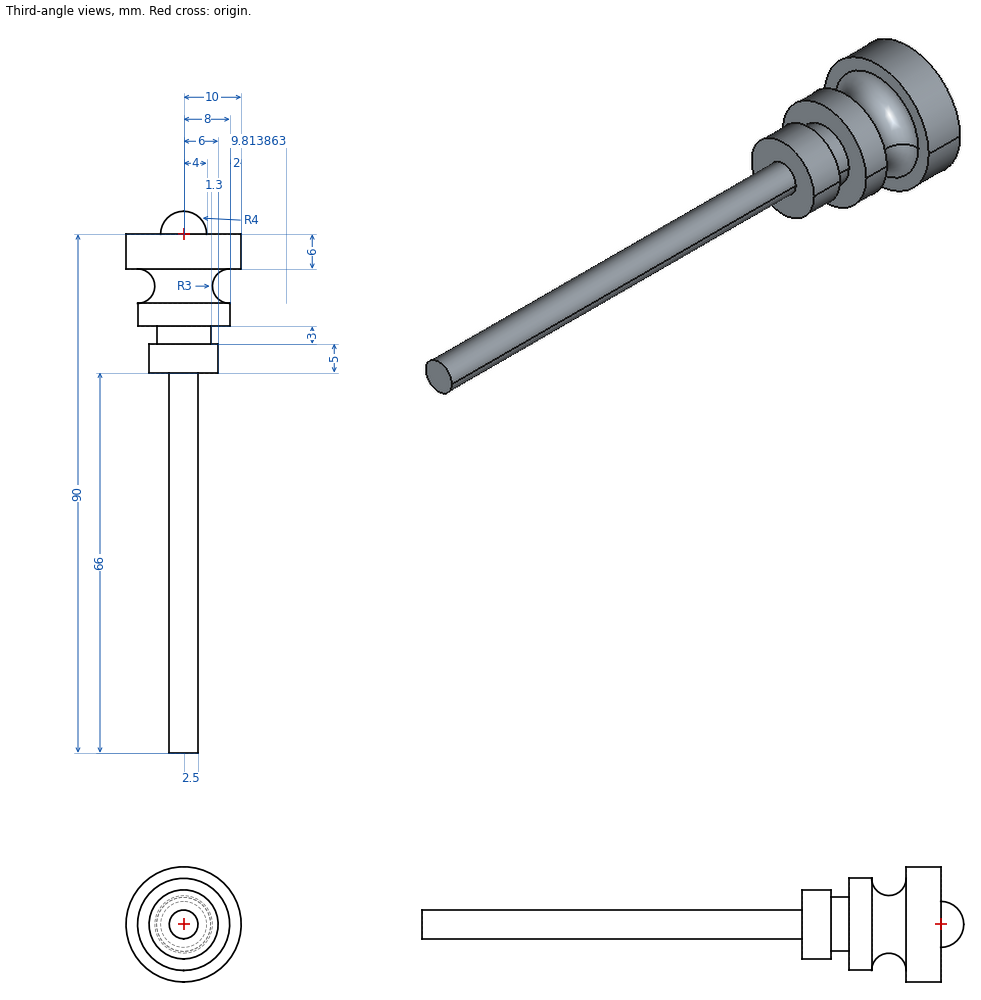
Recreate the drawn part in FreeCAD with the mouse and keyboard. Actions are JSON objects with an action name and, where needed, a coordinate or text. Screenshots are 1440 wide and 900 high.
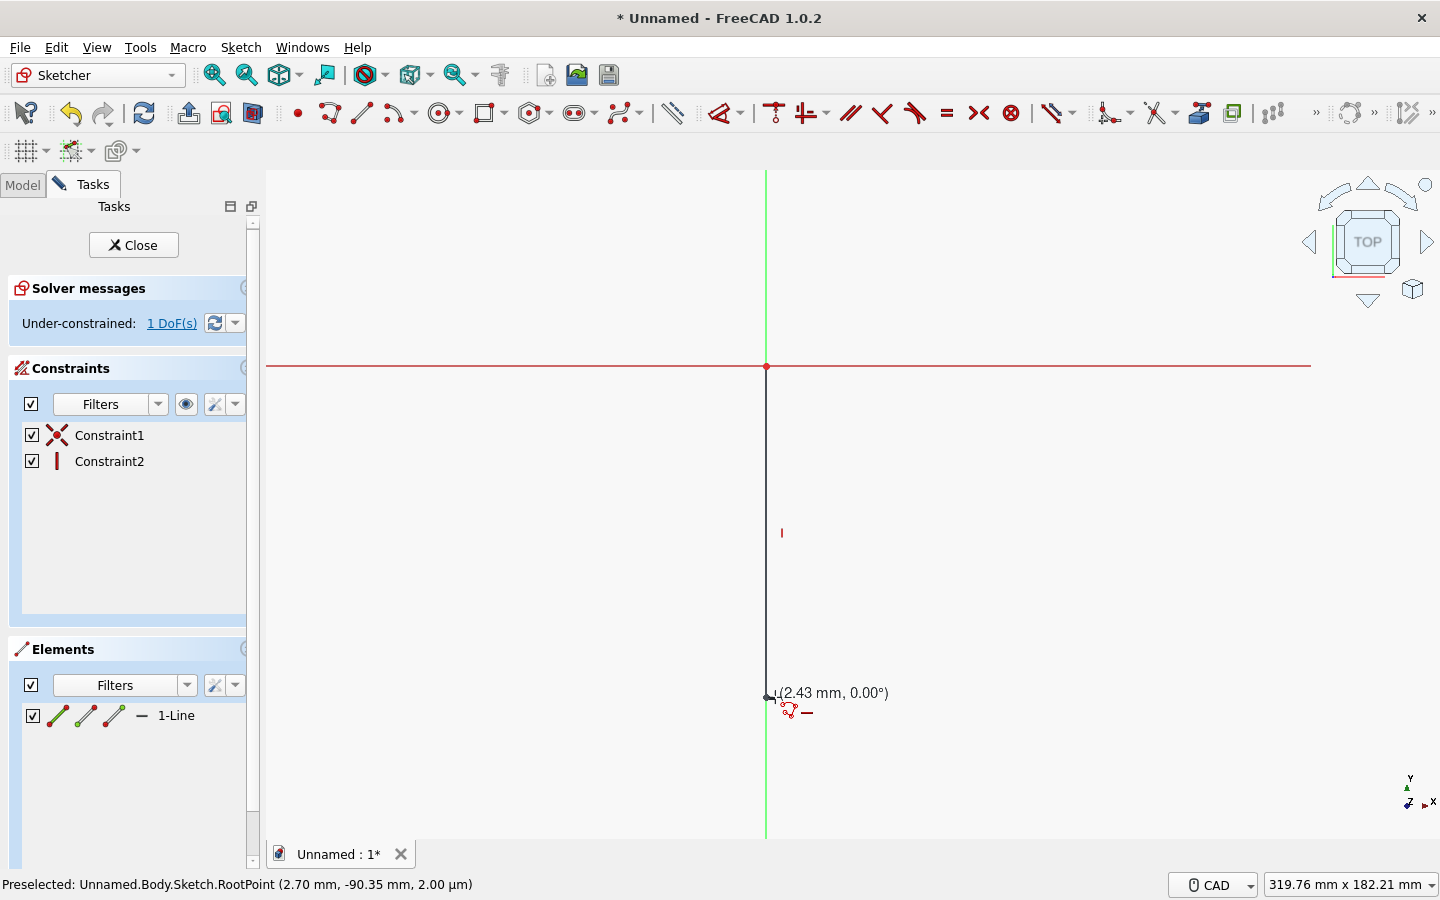
{"action": "scroll", "coordinate": [775, 697], "scroll_direction": "up", "scroll_amount": 3}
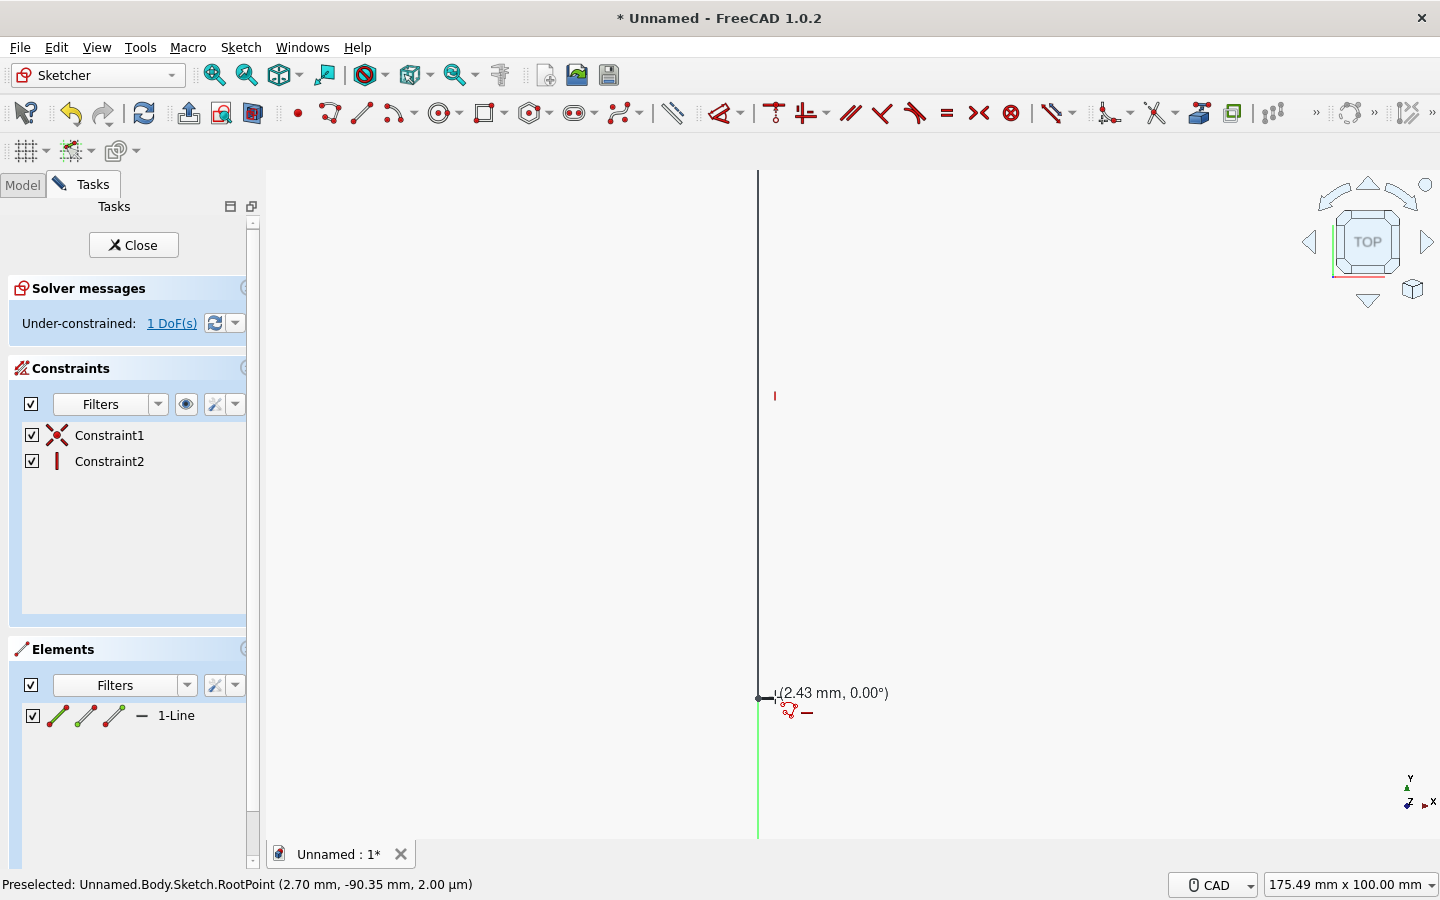
{"action": "left_click", "coordinate": [775, 696]}
{"action": "left_click", "coordinate": [775, 254]}
{"action": "left_click", "coordinate": [799, 254]}
{"action": "left_click", "coordinate": [799, 221]}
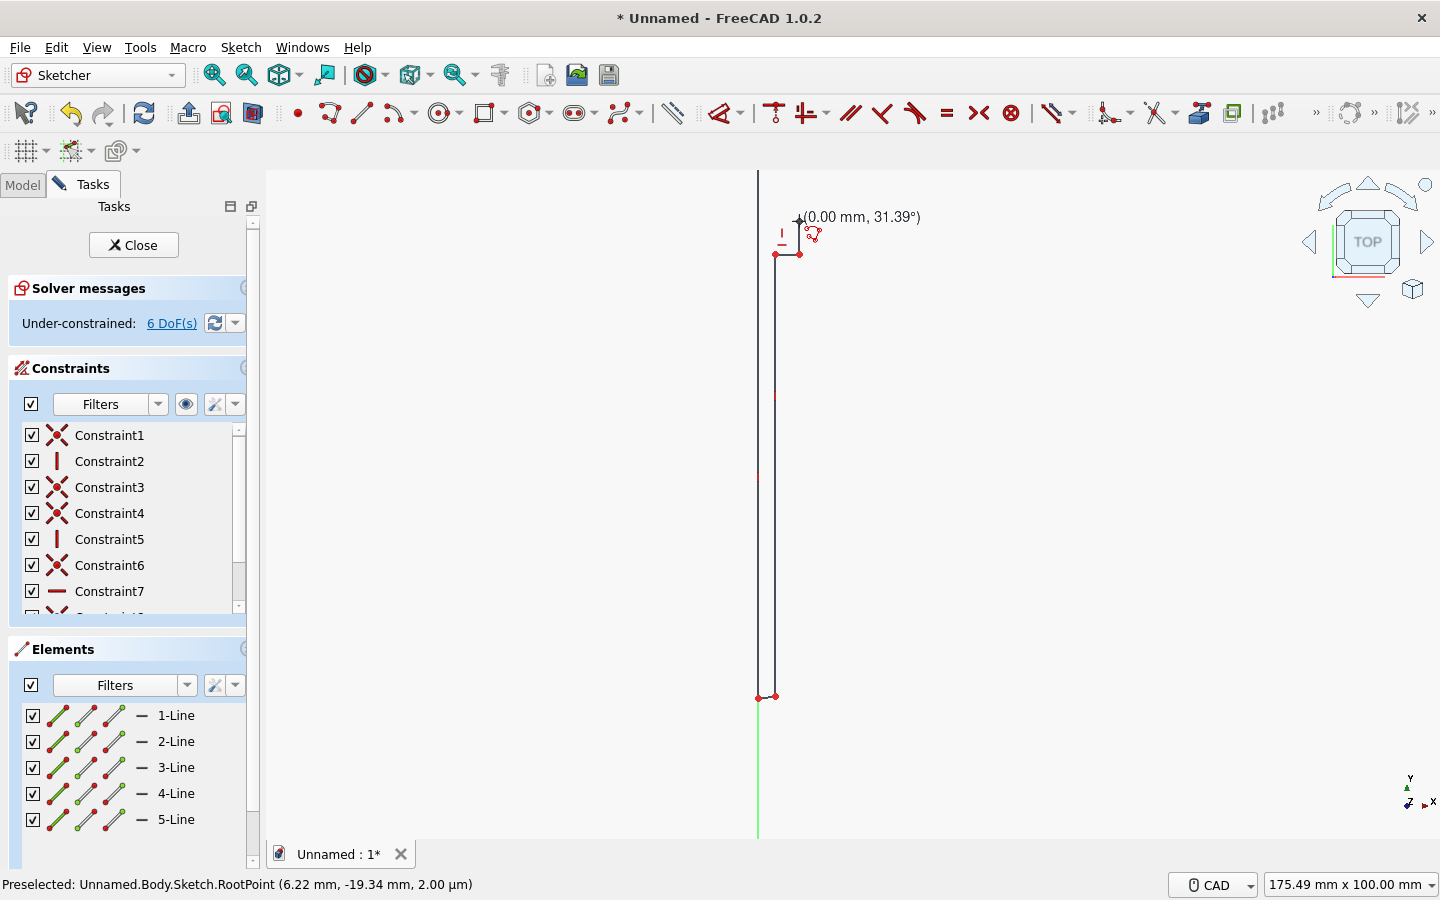
{"action": "scroll", "coordinate": [790, 221], "scroll_direction": "up", "scroll_amount": 4}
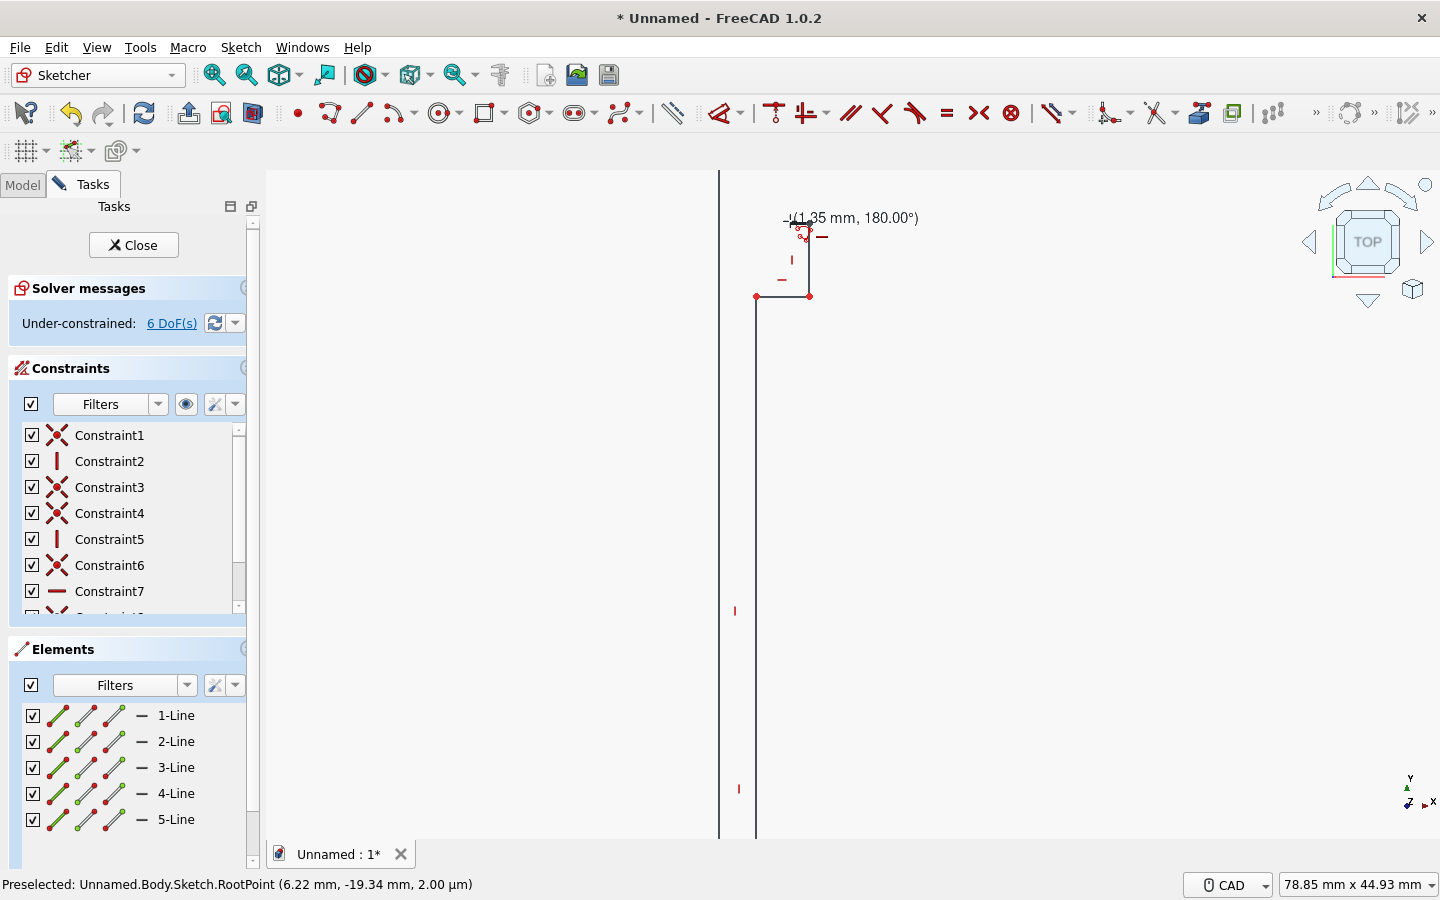
{"action": "left_click", "coordinate": [789, 221]}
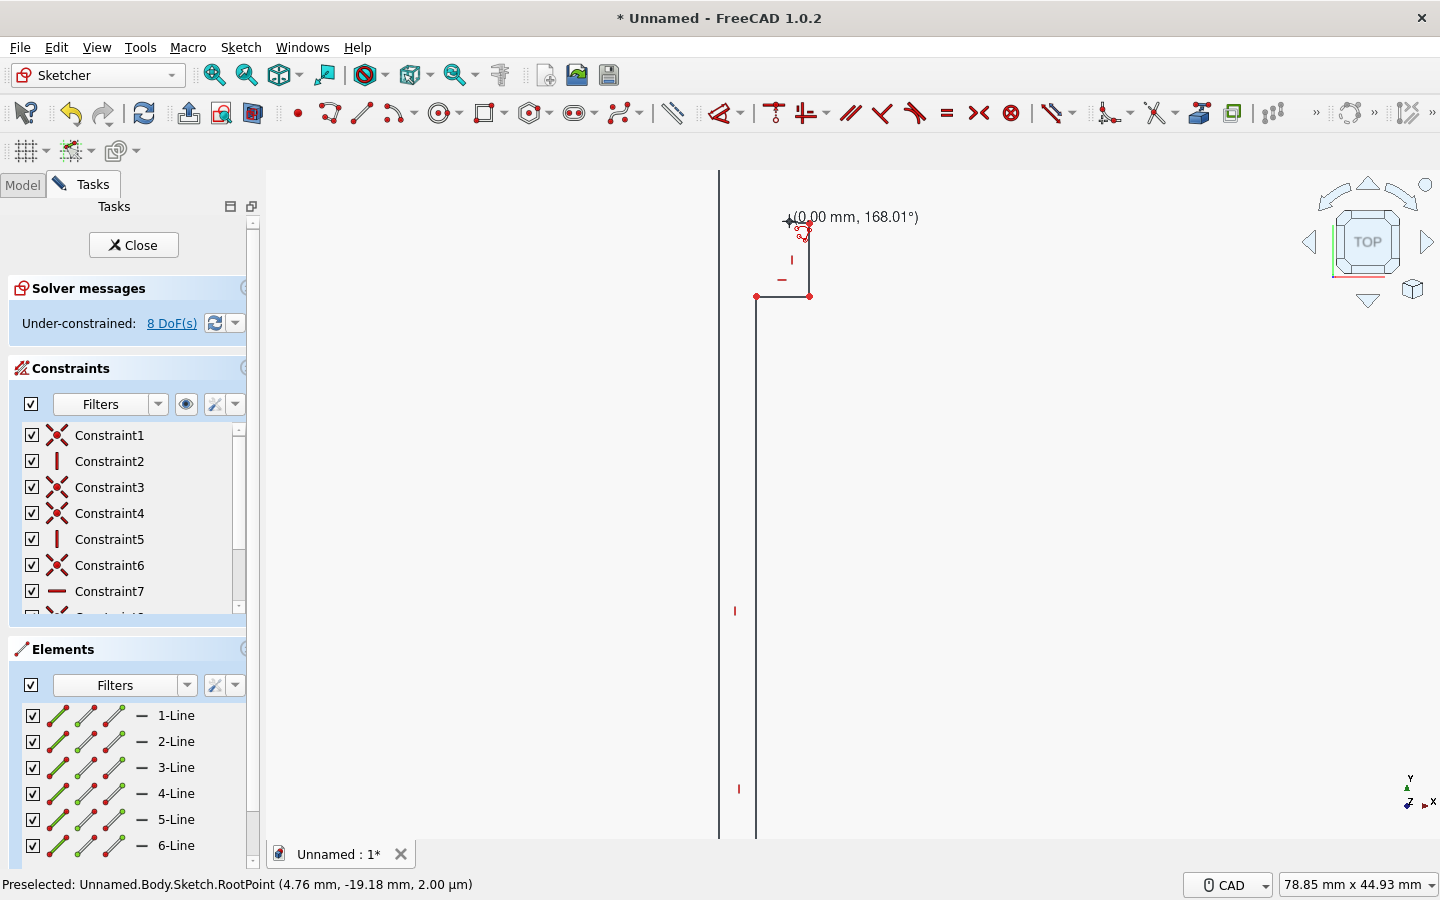
{"action": "scroll", "coordinate": [781, 460], "scroll_direction": "down", "scroll_amount": 6}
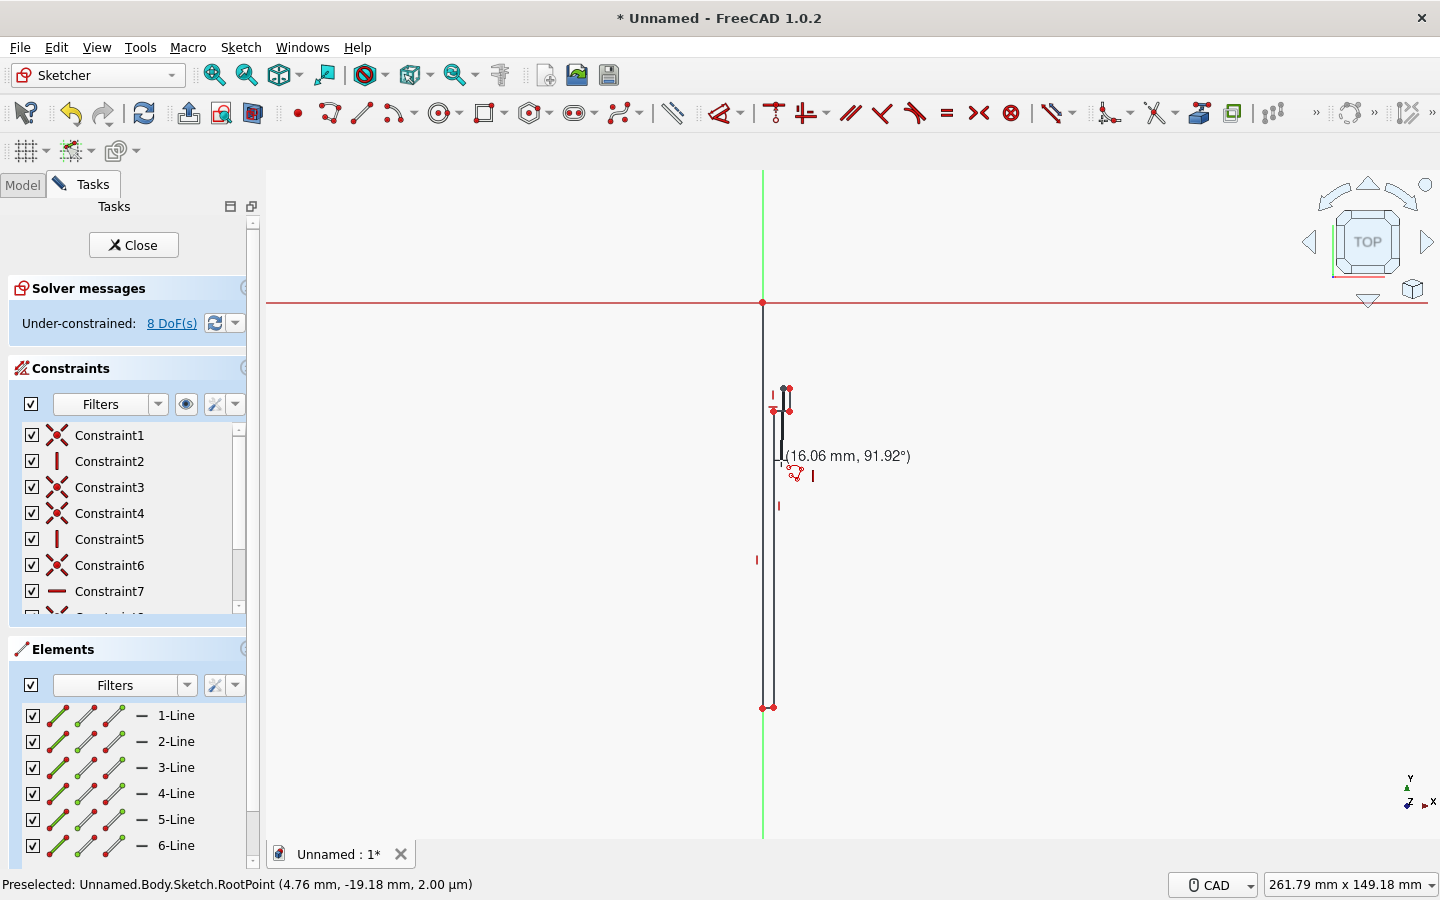
{"action": "left_click", "coordinate": [784, 375]}
{"action": "left_click", "coordinate": [799, 375]}
{"action": "left_click", "coordinate": [799, 330]}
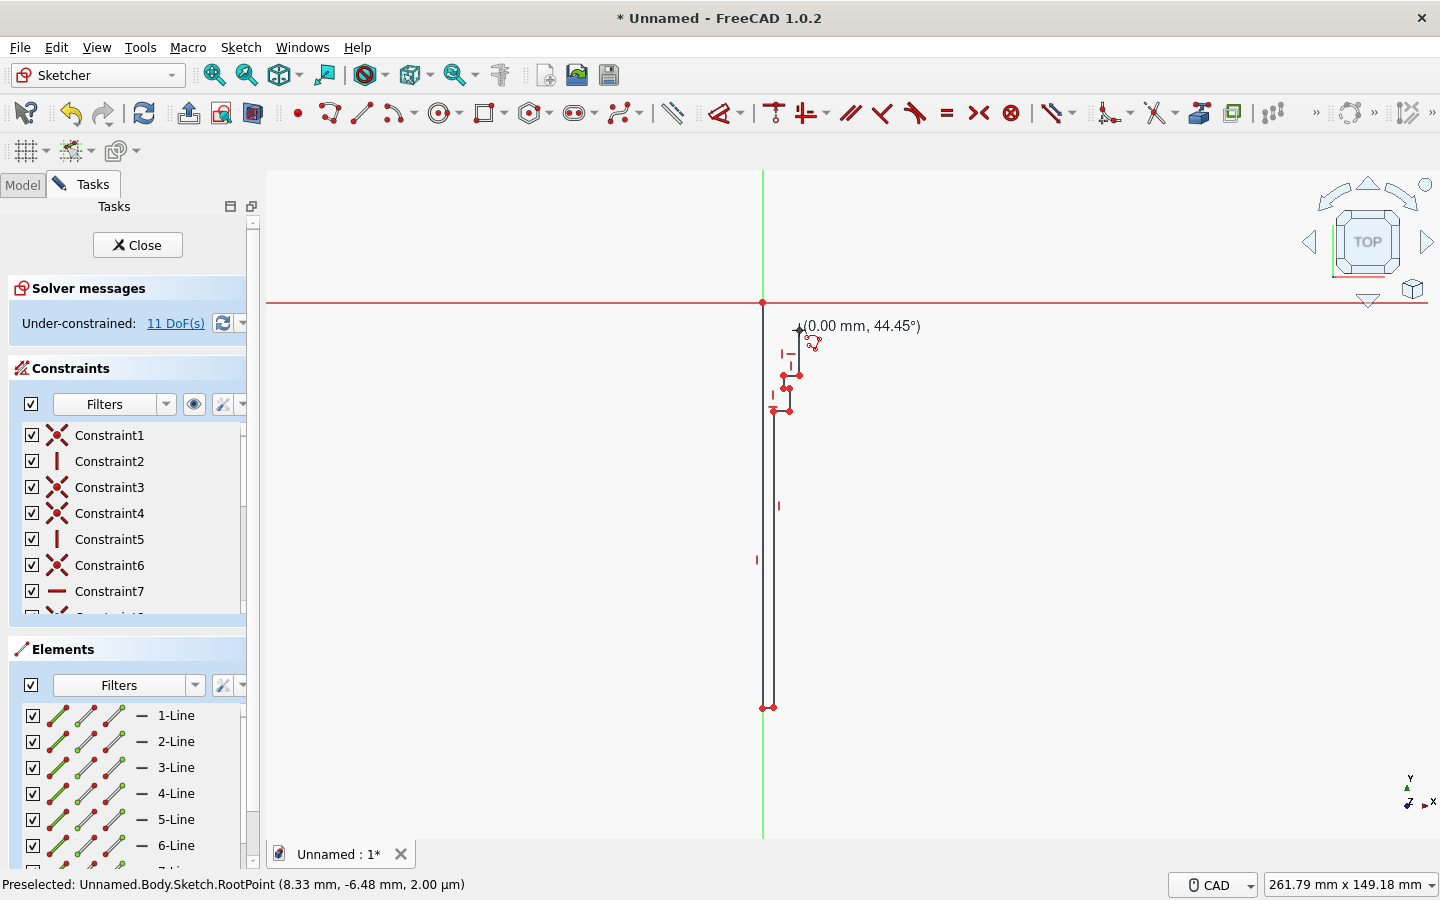
{"action": "scroll", "coordinate": [807, 330], "scroll_direction": "up", "scroll_amount": 3}